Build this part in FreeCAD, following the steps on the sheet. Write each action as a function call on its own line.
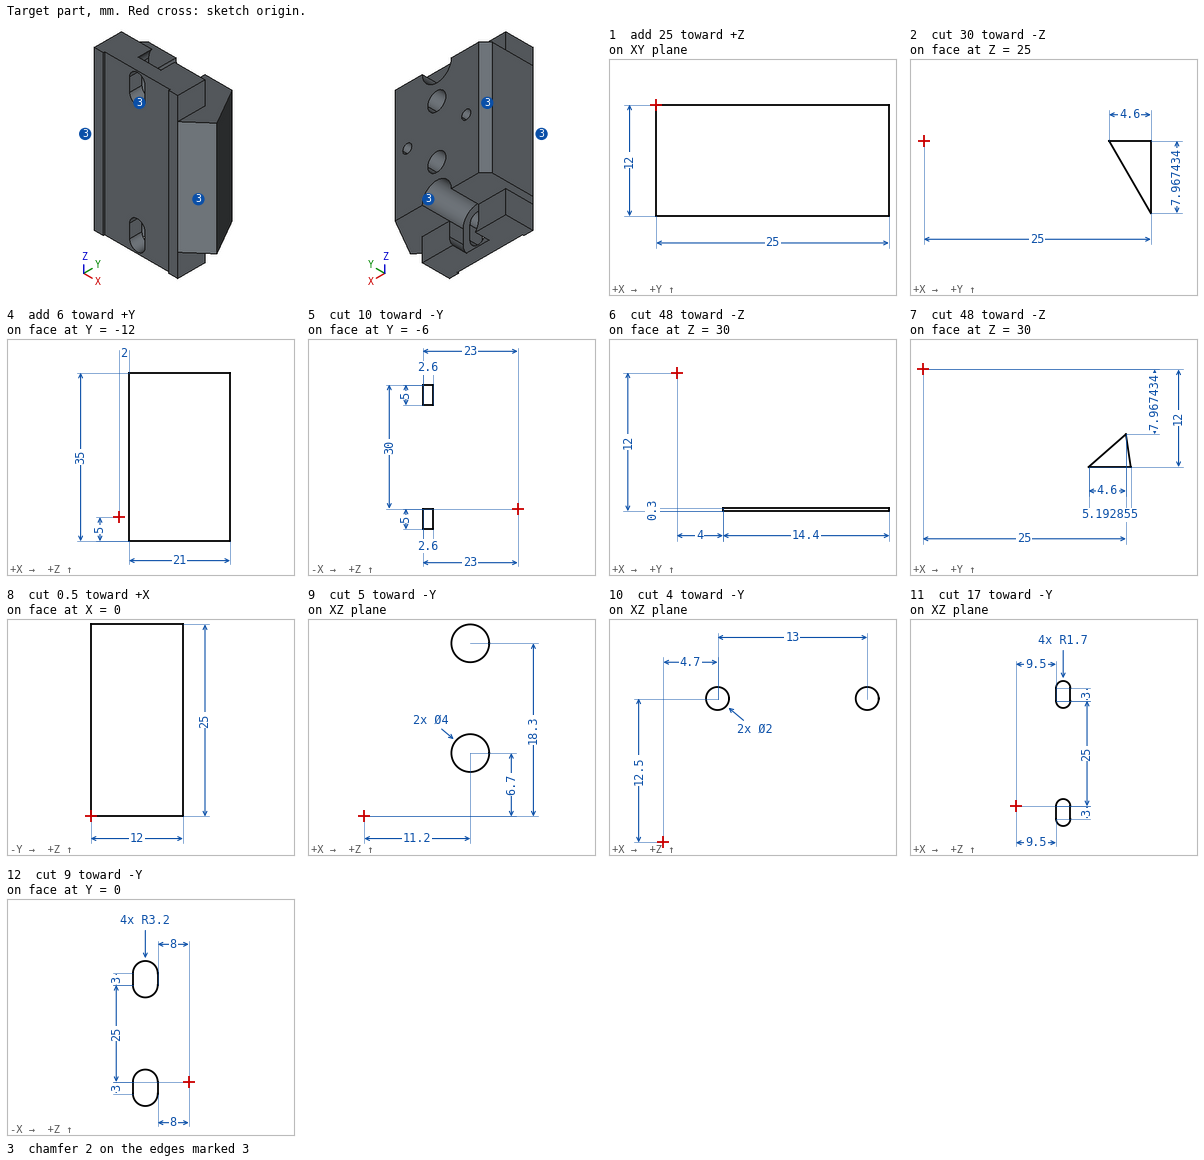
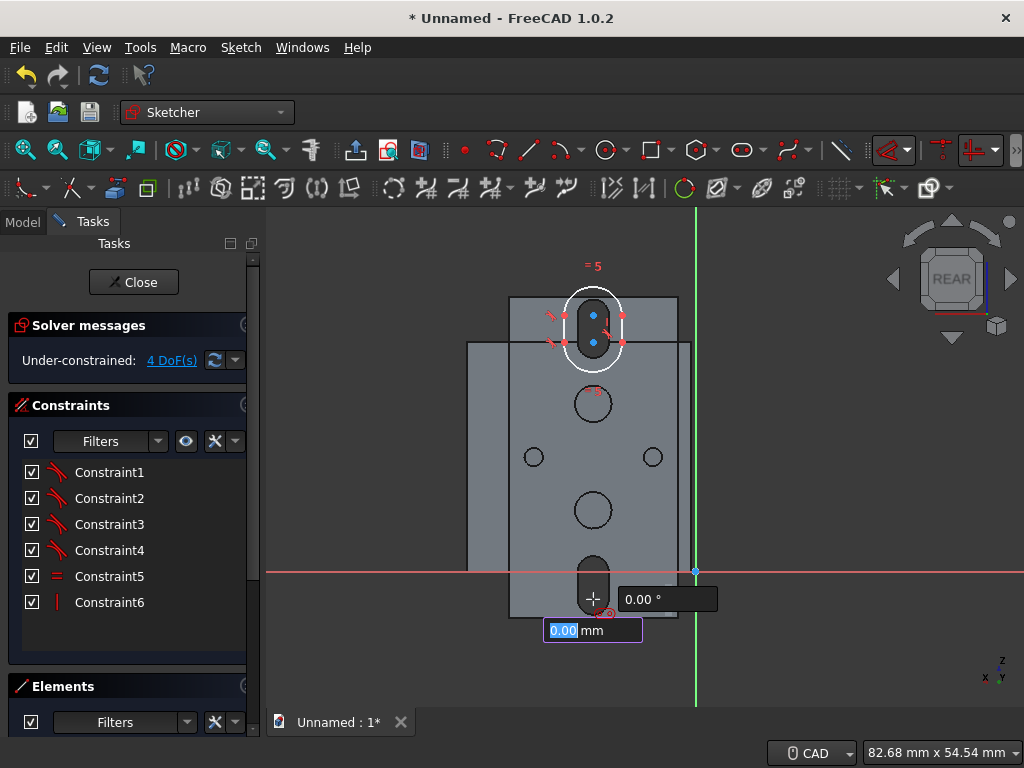
click(593, 572)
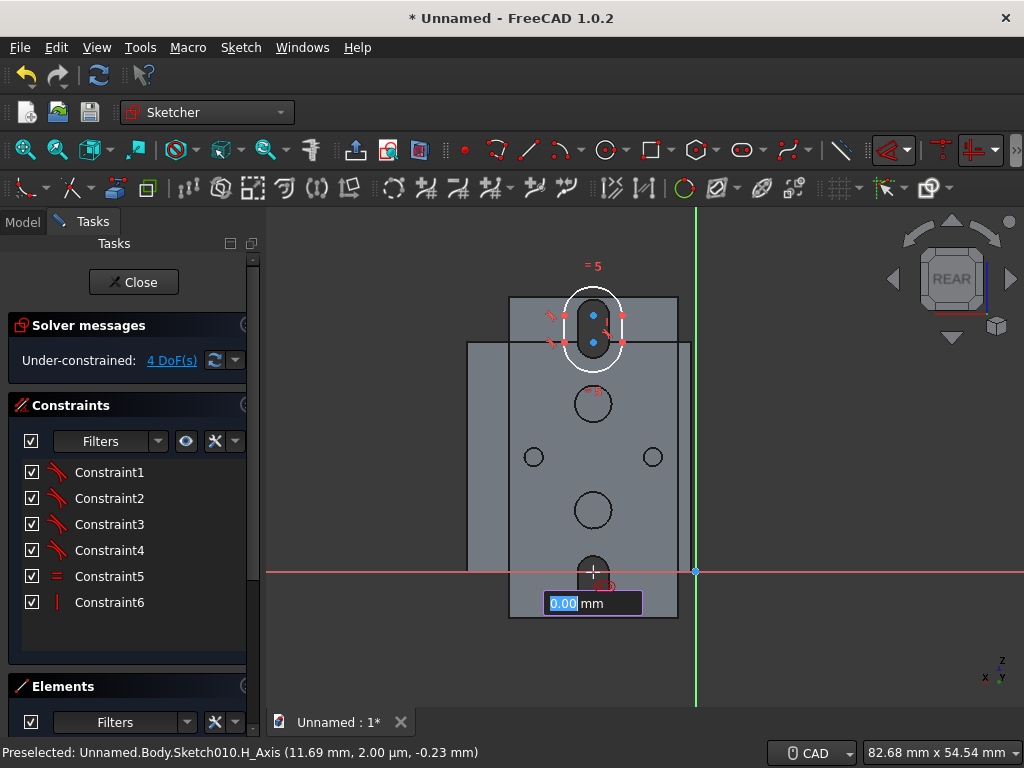
click(564, 590)
key(Escape)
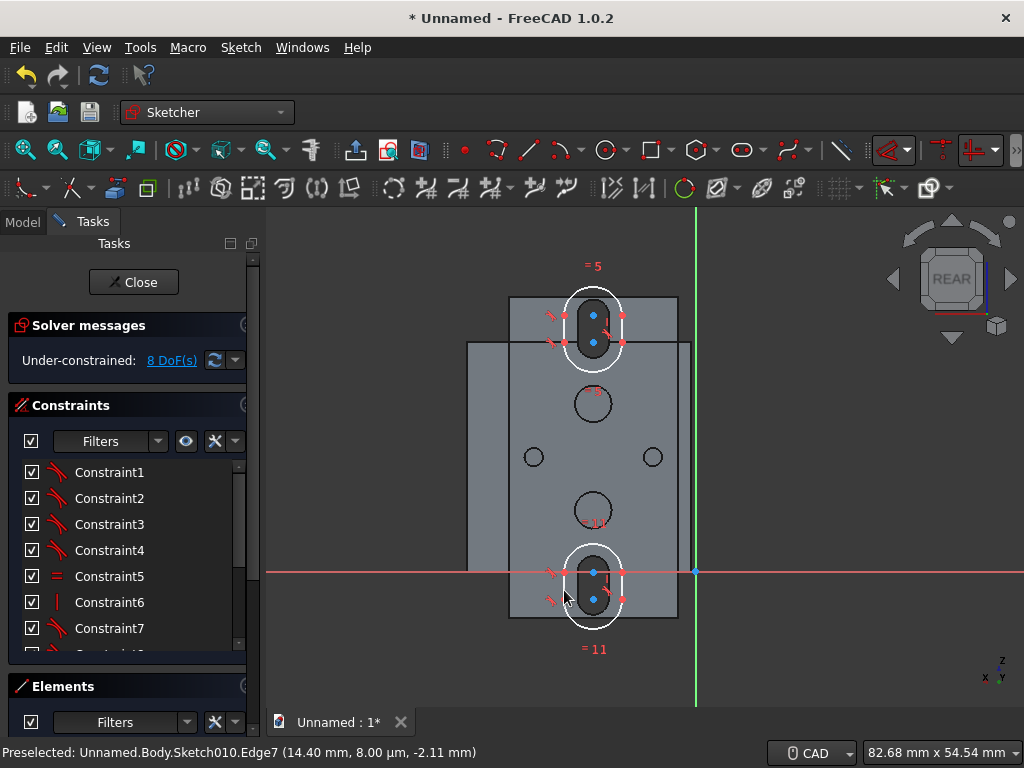
click(576, 366)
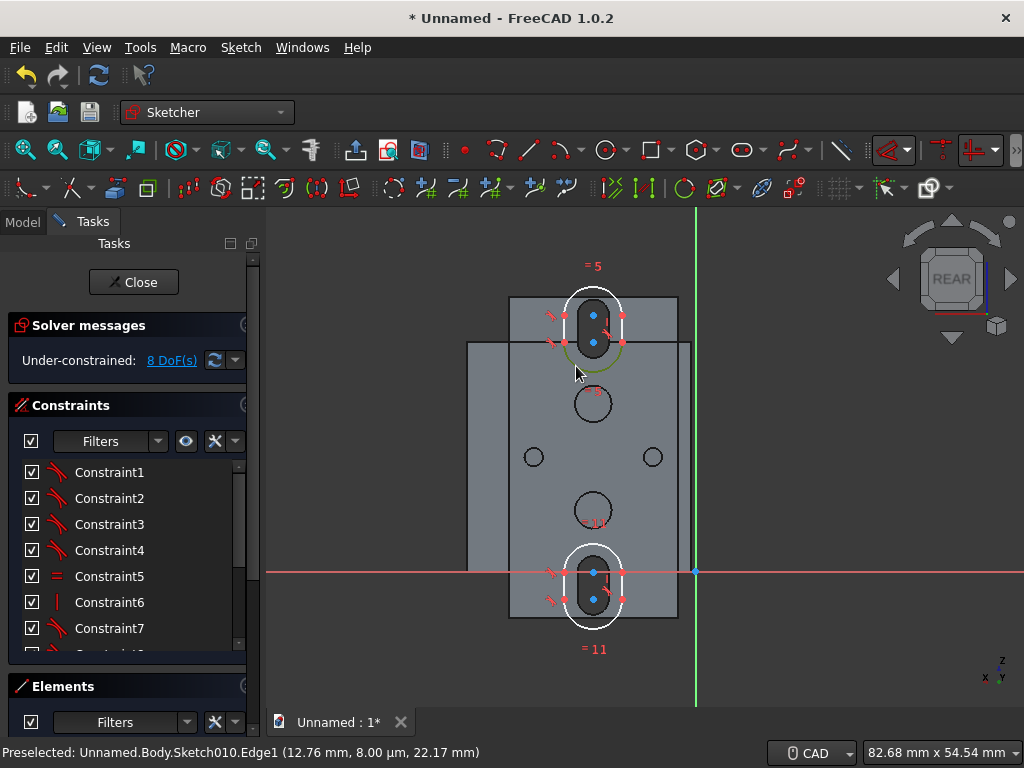
click(576, 623)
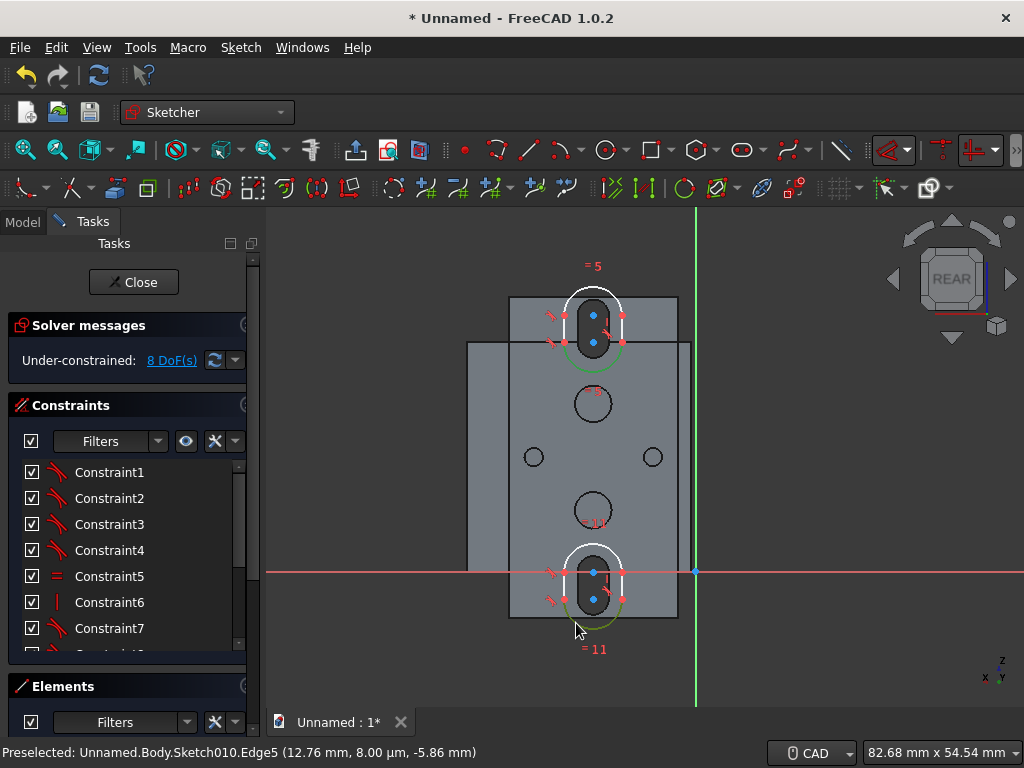
key(e)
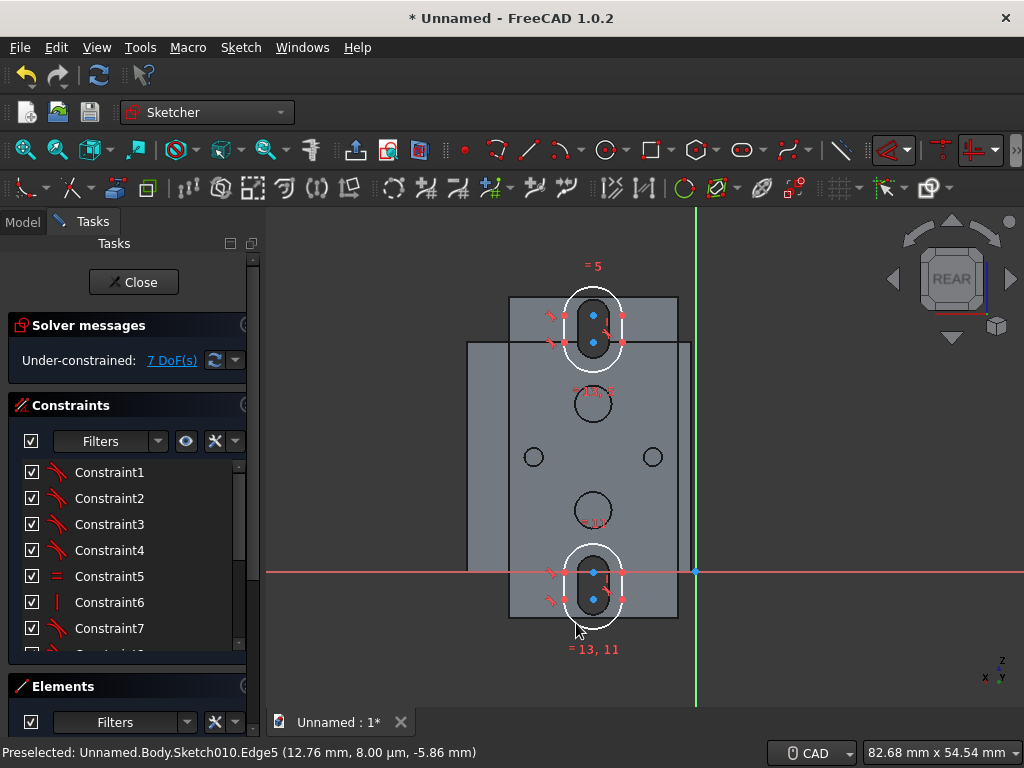
click(593, 573)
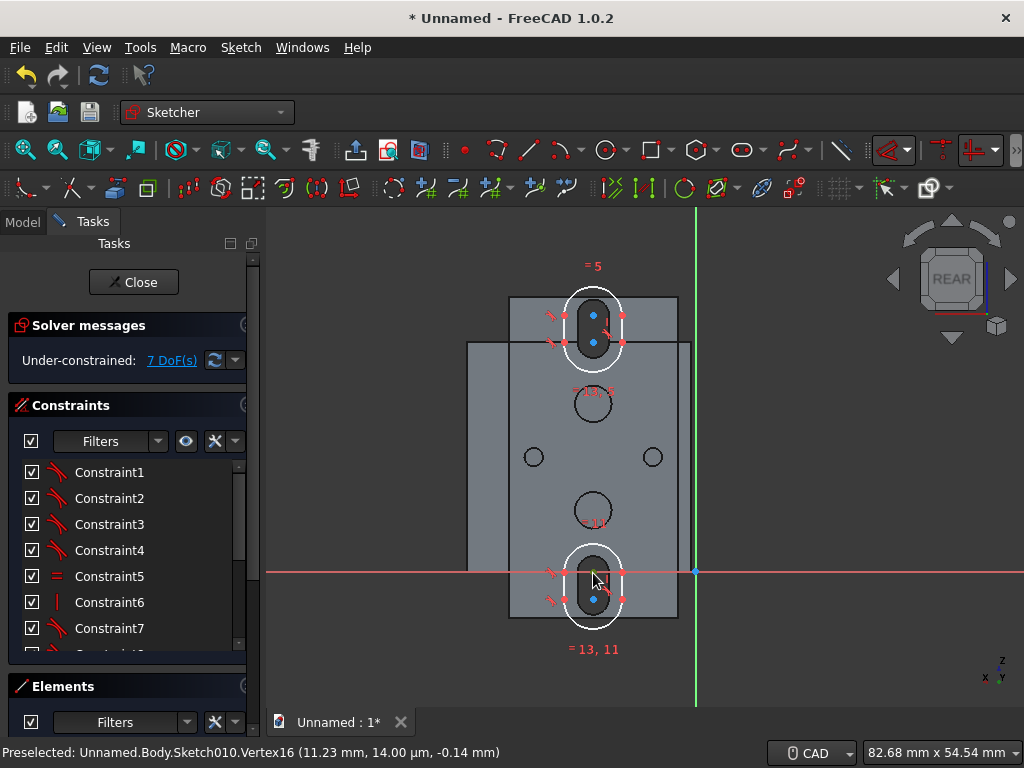
click(334, 572)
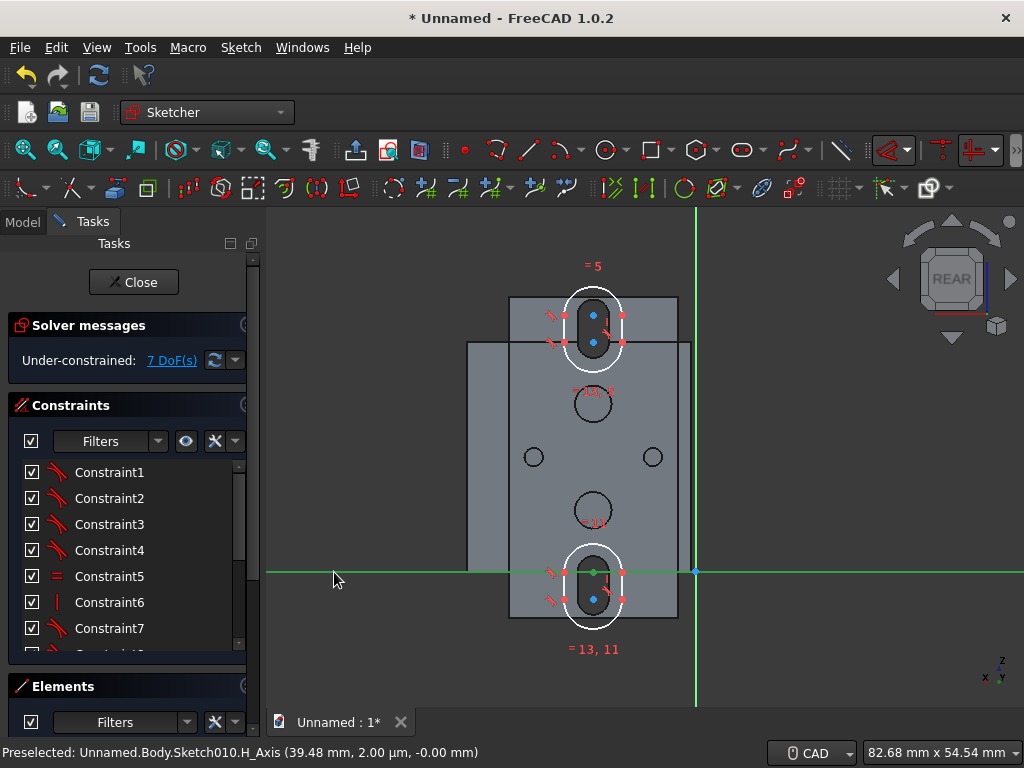
click(942, 150)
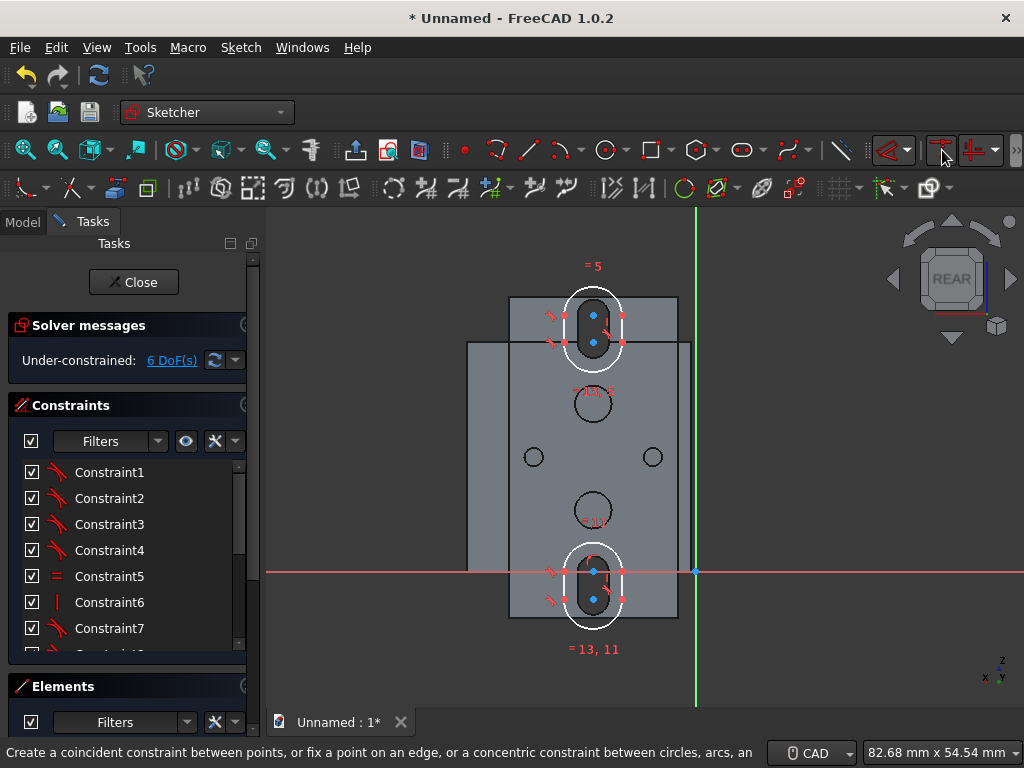
scroll(576, 366, up, 2)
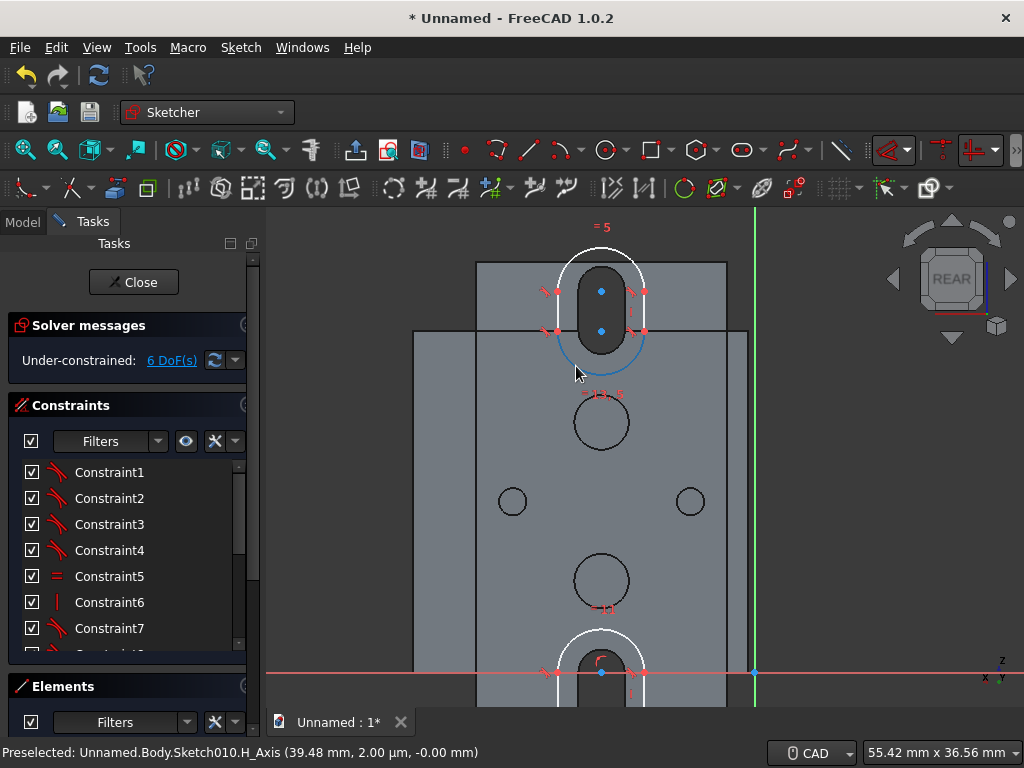
click(576, 367)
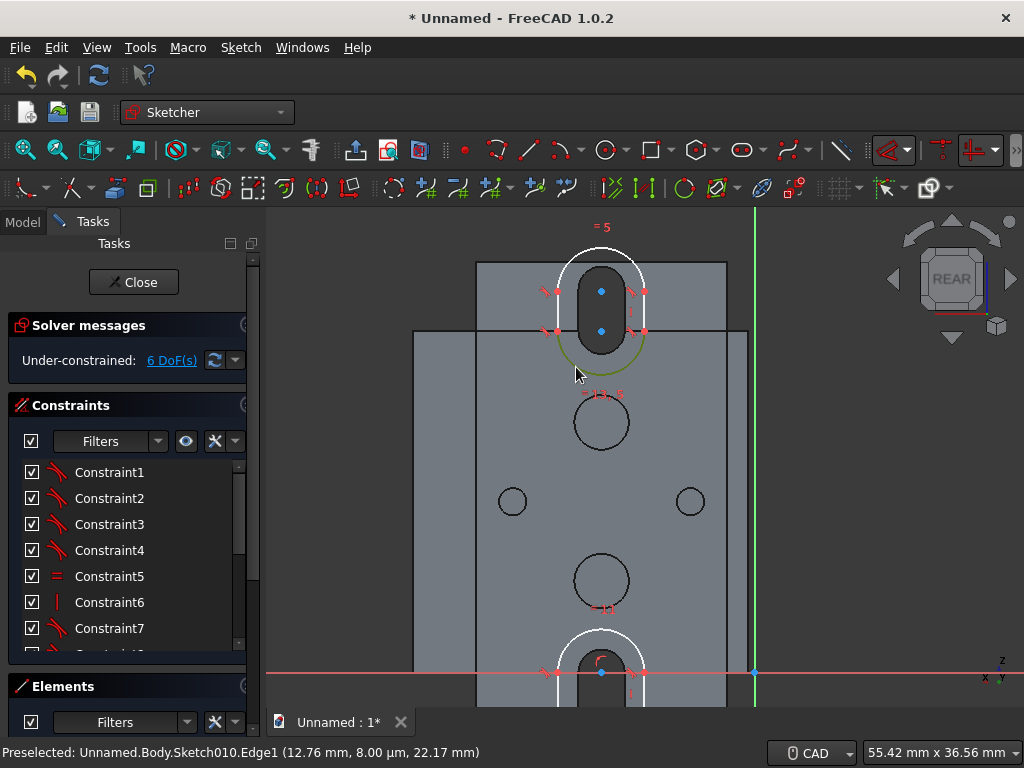
key(k)
key(r)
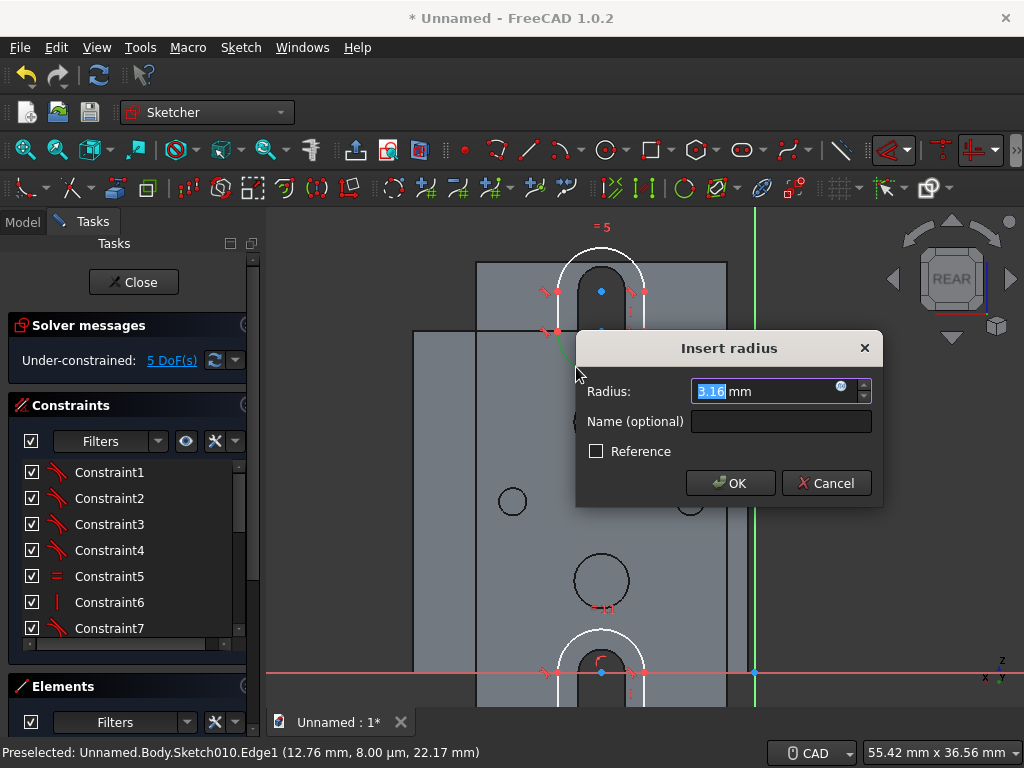
text(3.2)
key(Return)